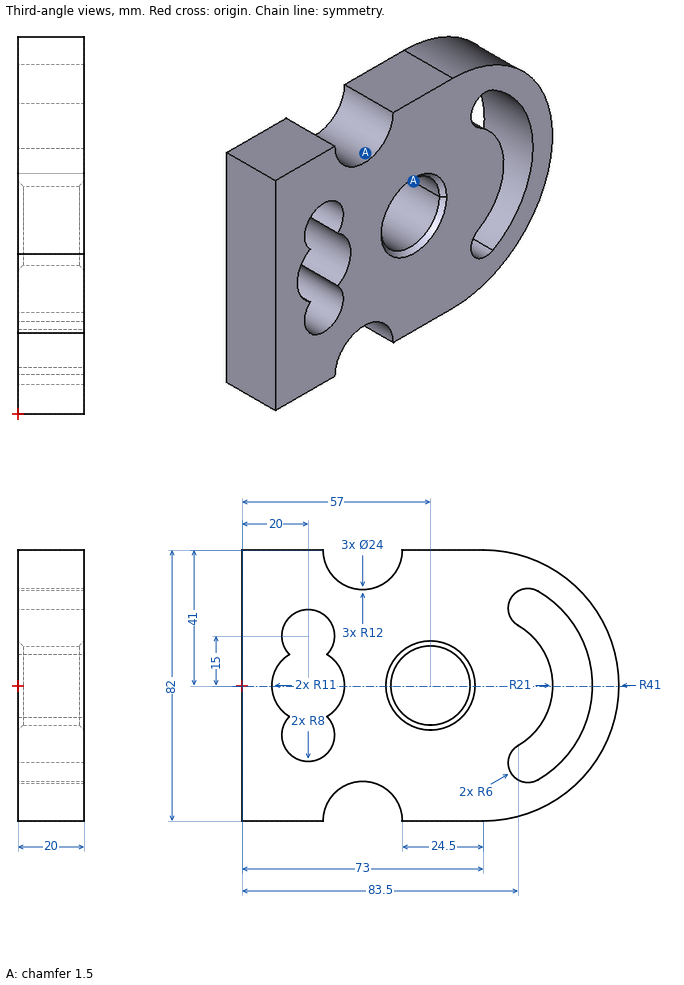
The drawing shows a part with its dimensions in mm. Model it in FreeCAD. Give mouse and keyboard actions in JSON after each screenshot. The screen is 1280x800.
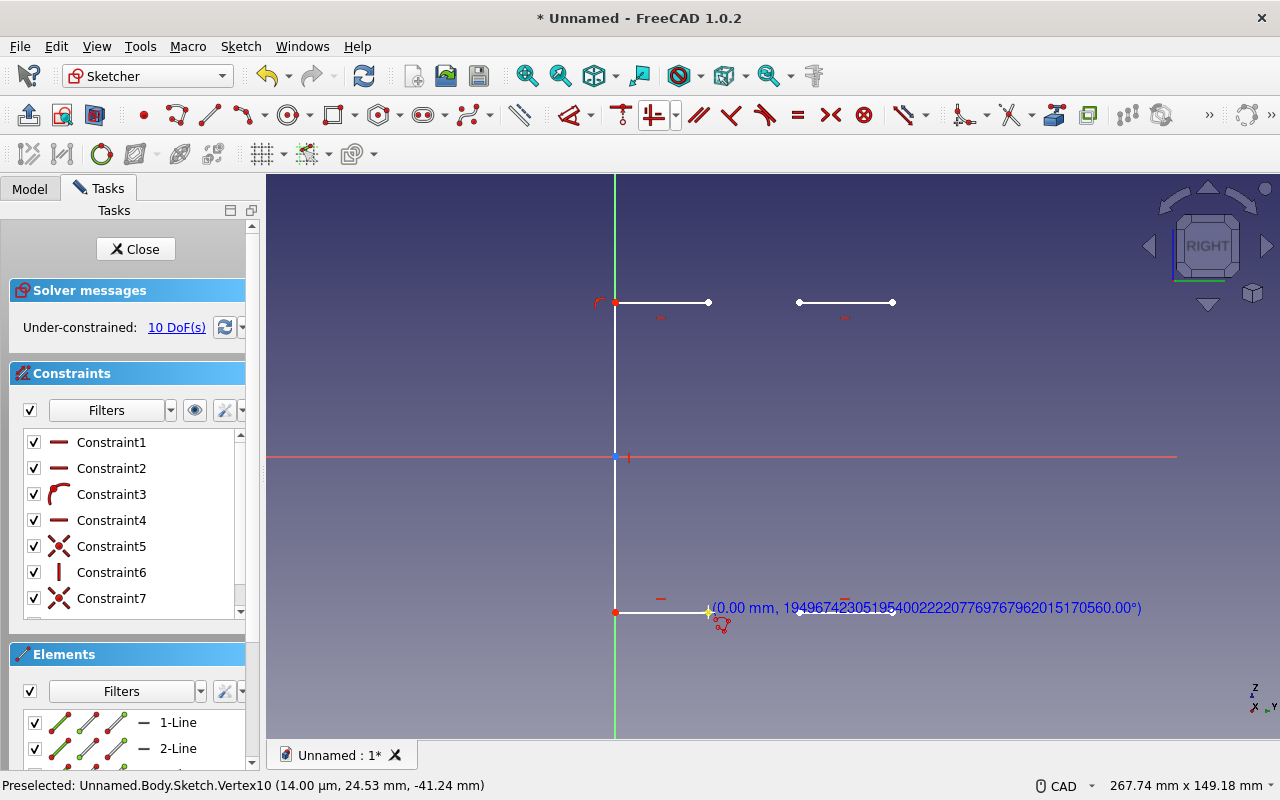
{"action": "key", "text": "g 3 a"}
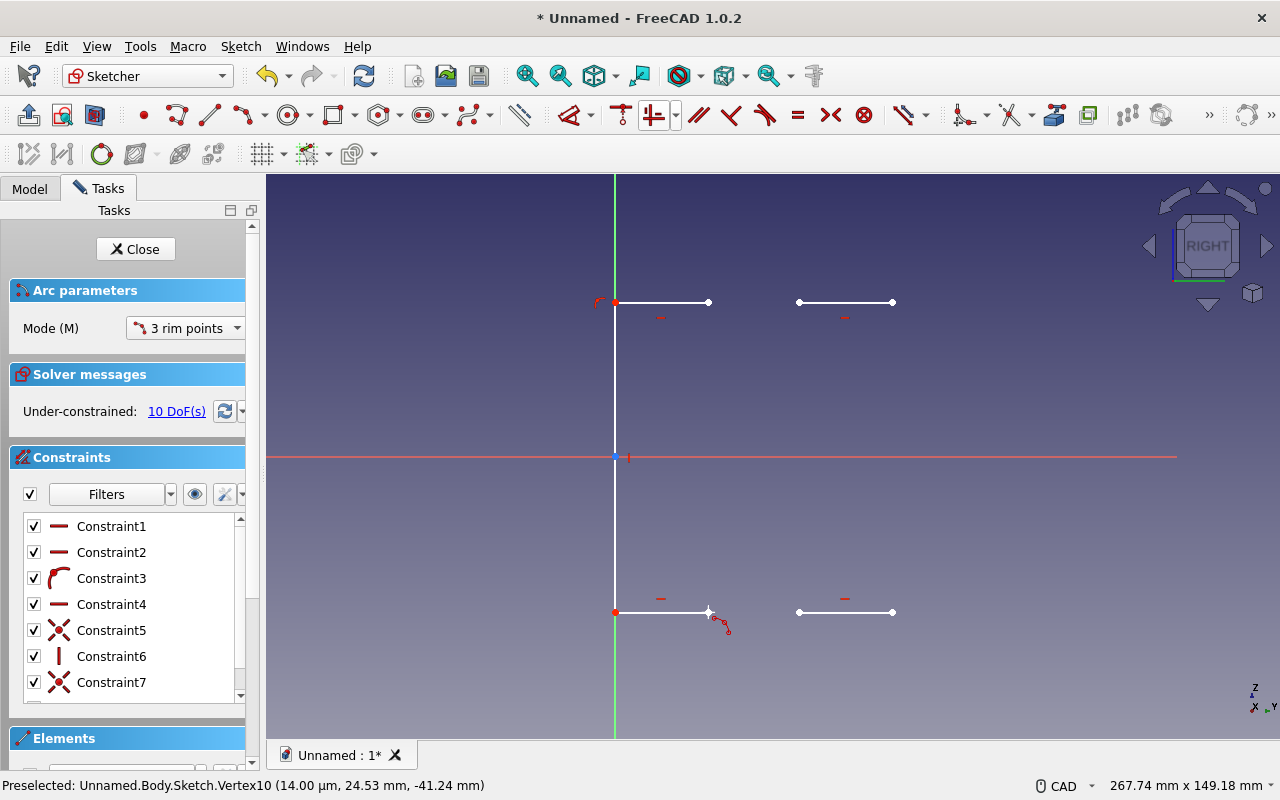
{"action": "left_click", "coordinate": [892, 613]}
{"action": "left_click", "coordinate": [892, 303]}
{"action": "left_click", "coordinate": [1039, 505]}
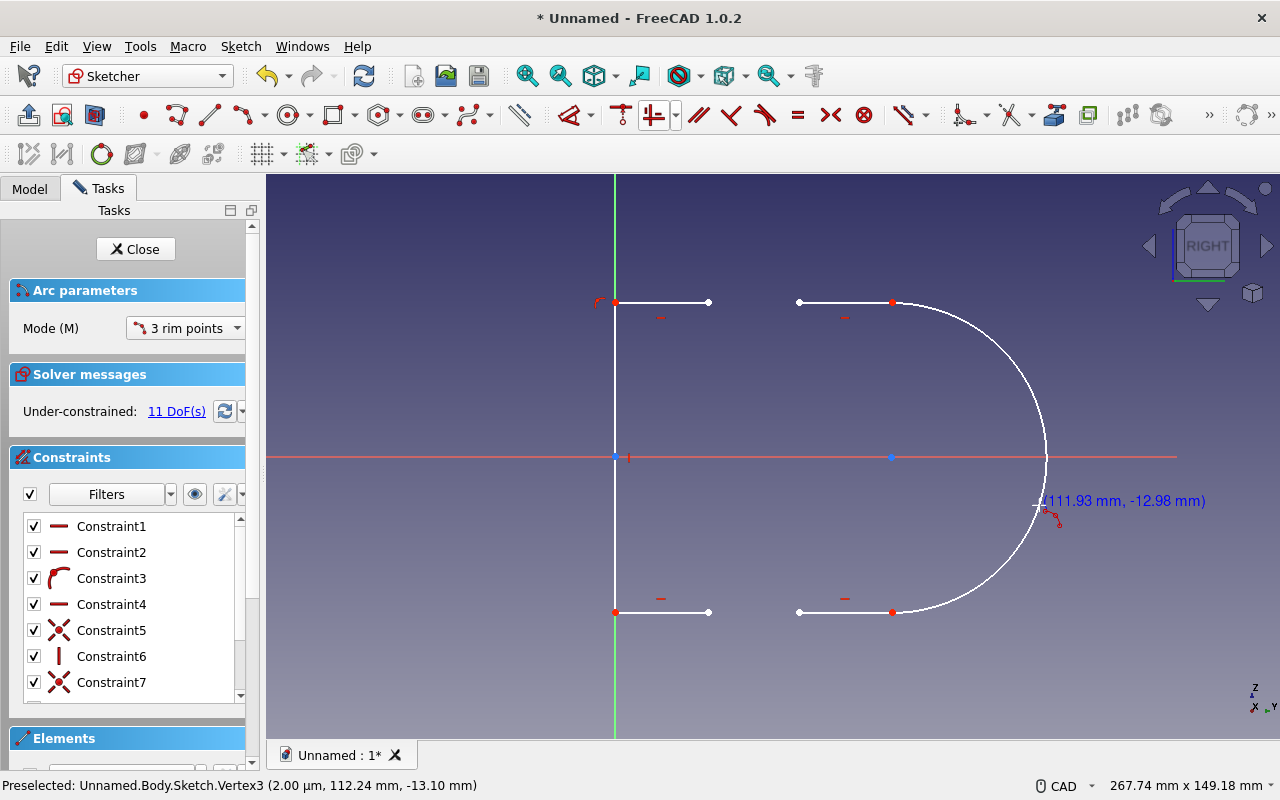
{"action": "left_click", "coordinate": [799, 303]}
{"action": "left_click", "coordinate": [708, 303]}
{"action": "left_click", "coordinate": [753, 347]}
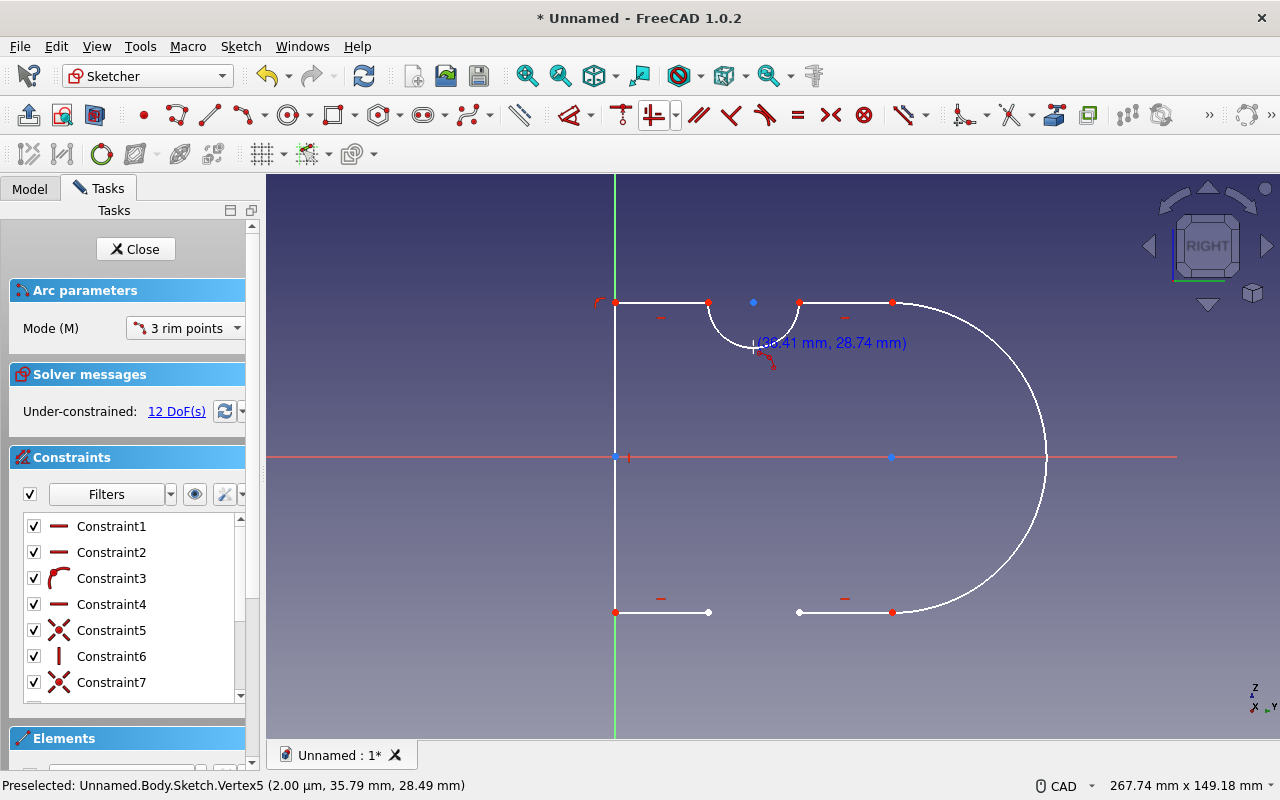
{"action": "left_click", "coordinate": [708, 613]}
{"action": "left_click", "coordinate": [799, 613]}
{"action": "left_click", "coordinate": [753, 567]}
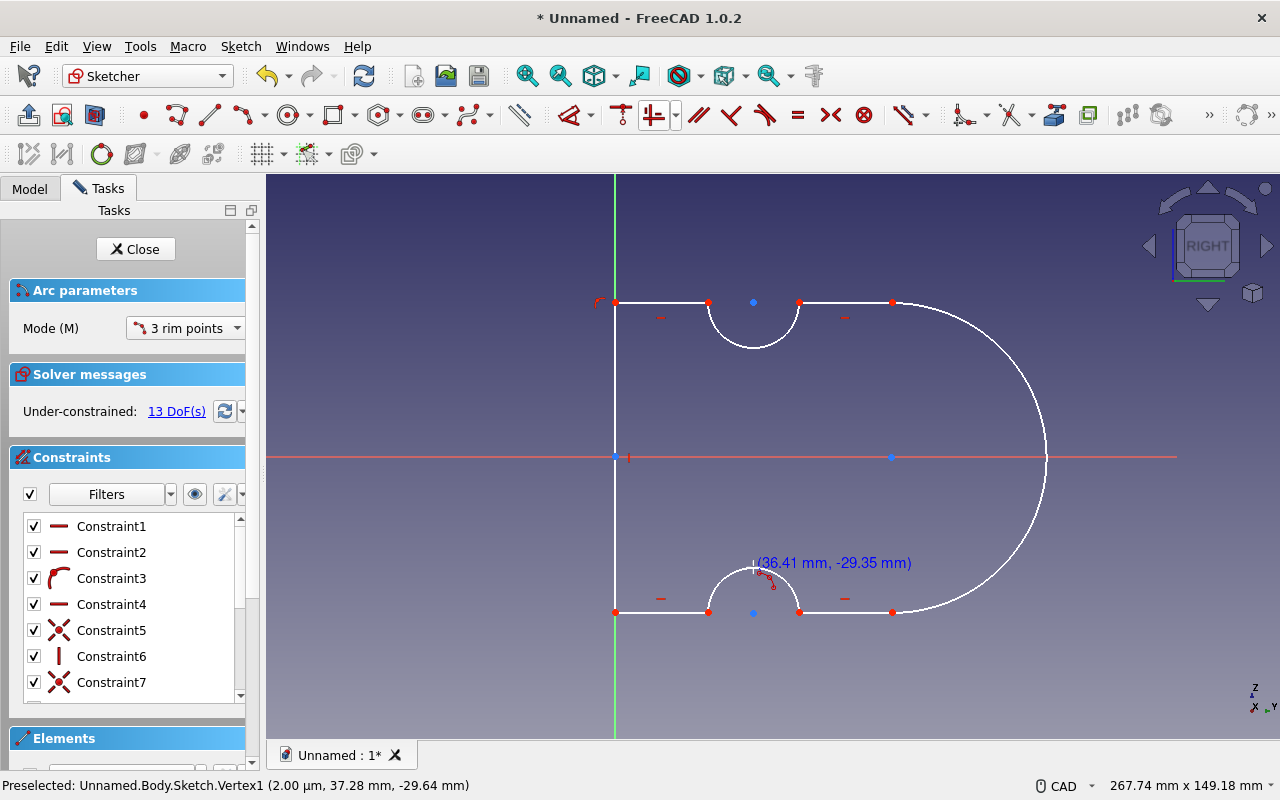
{"action": "left_click", "coordinate": [669, 492]}
{"action": "left_click", "coordinate": [669, 421]}
{"action": "left_click", "coordinate": [653, 440]}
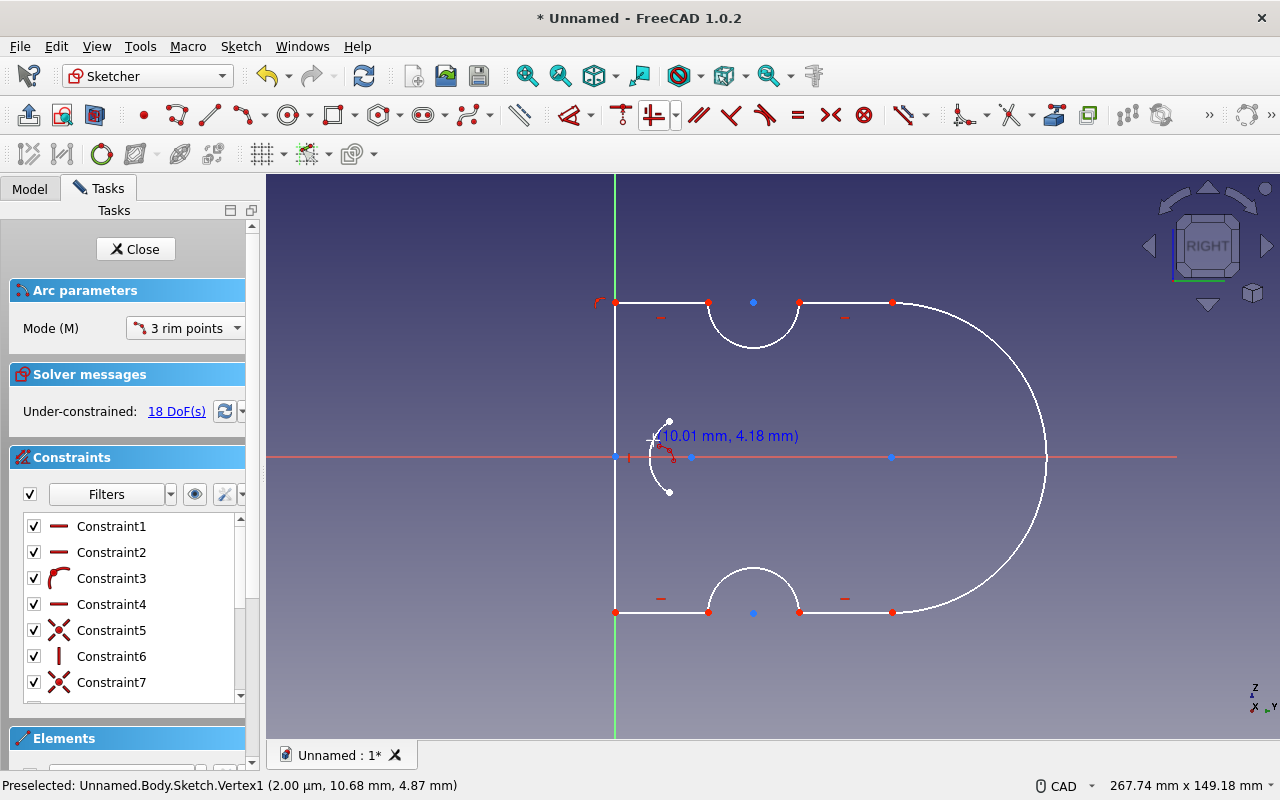
{"action": "left_click", "coordinate": [669, 422]}
{"action": "left_click", "coordinate": [712, 421]}
{"action": "left_click", "coordinate": [691, 370]}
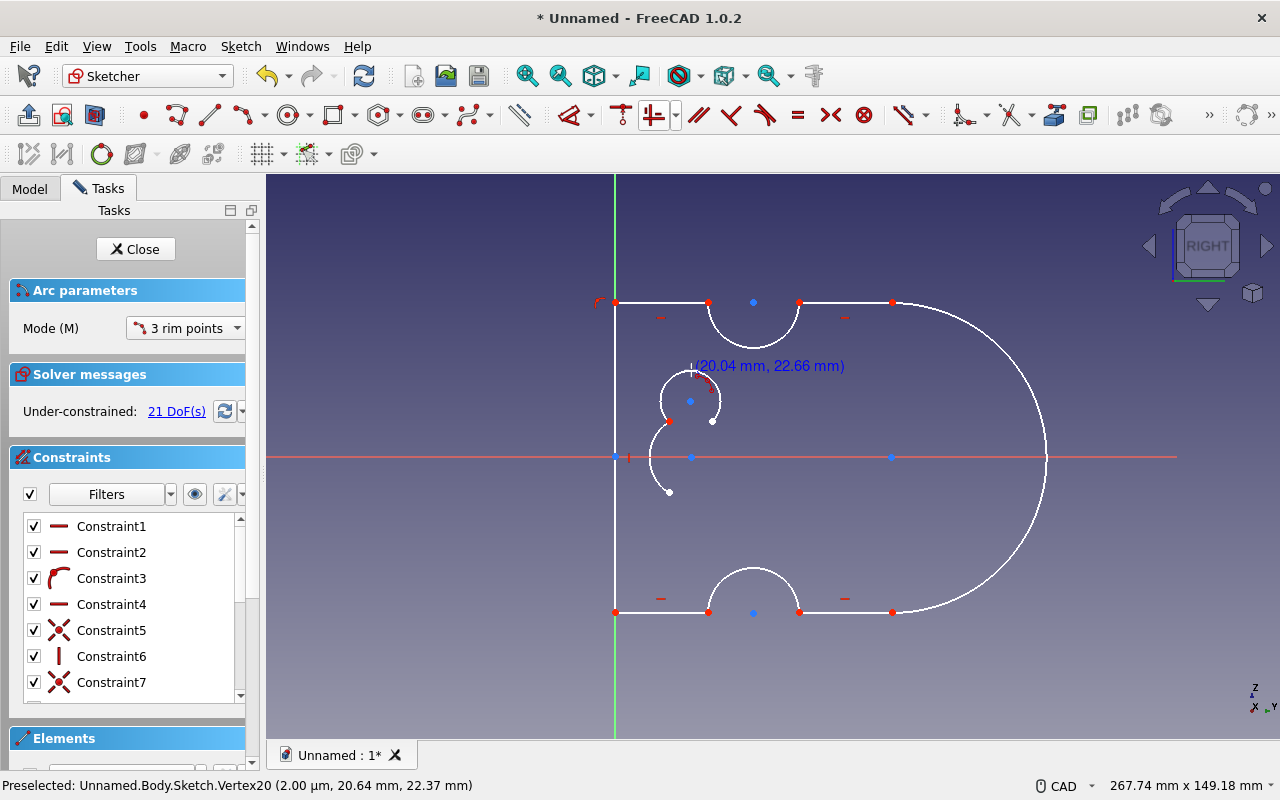
{"action": "left_click", "coordinate": [712, 422]}
{"action": "left_click", "coordinate": [712, 492]}
{"action": "left_click", "coordinate": [729, 473]}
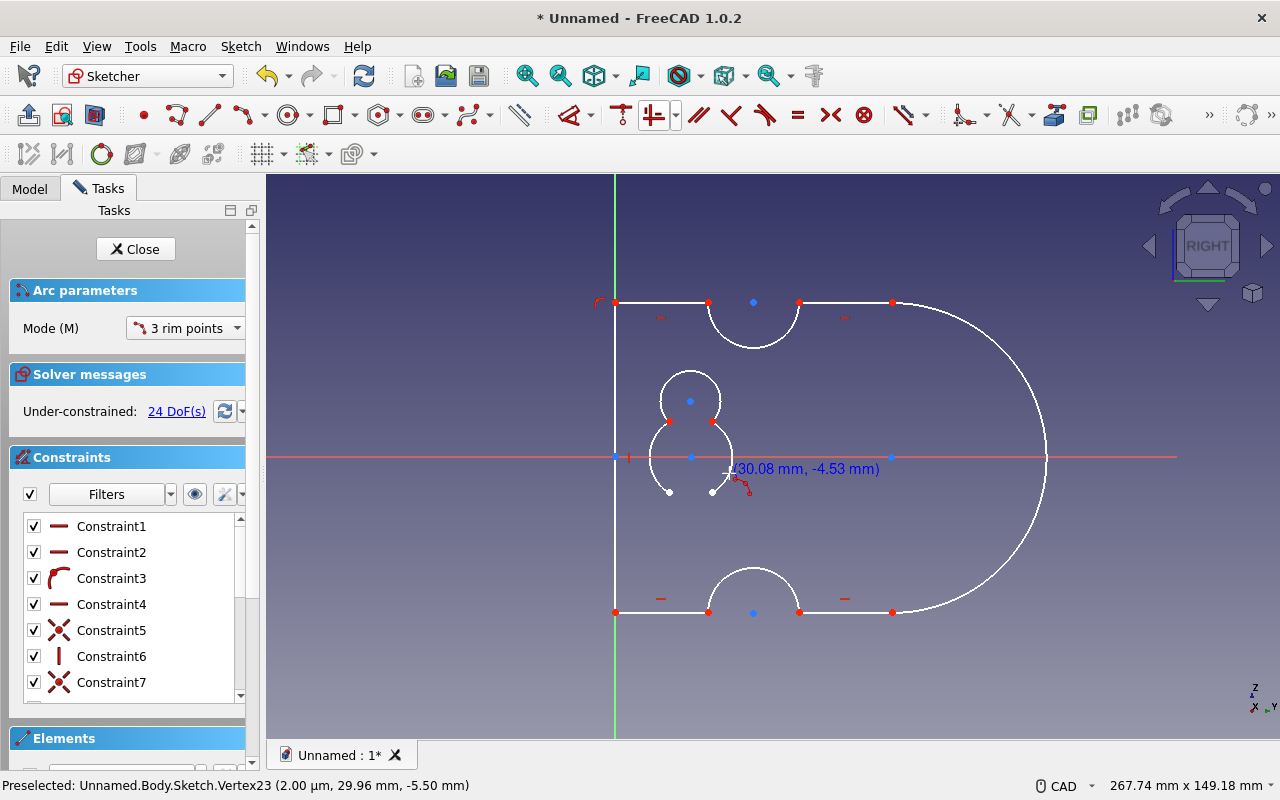
{"action": "left_click", "coordinate": [712, 493]}
{"action": "left_click", "coordinate": [669, 493]}
{"action": "left_click", "coordinate": [691, 544]}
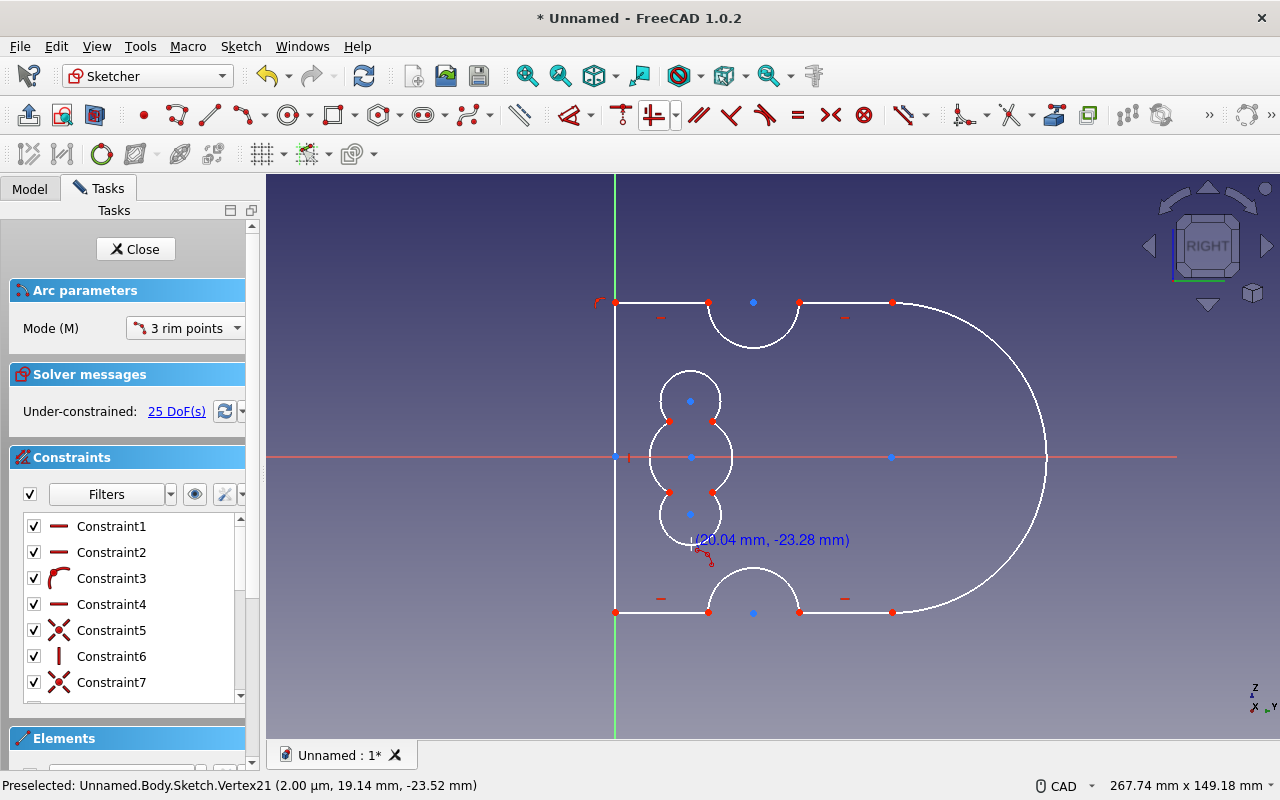
{"action": "left_click", "coordinate": [931, 526]}
{"action": "left_click", "coordinate": [931, 388]}
{"action": "left_click", "coordinate": [969, 473]}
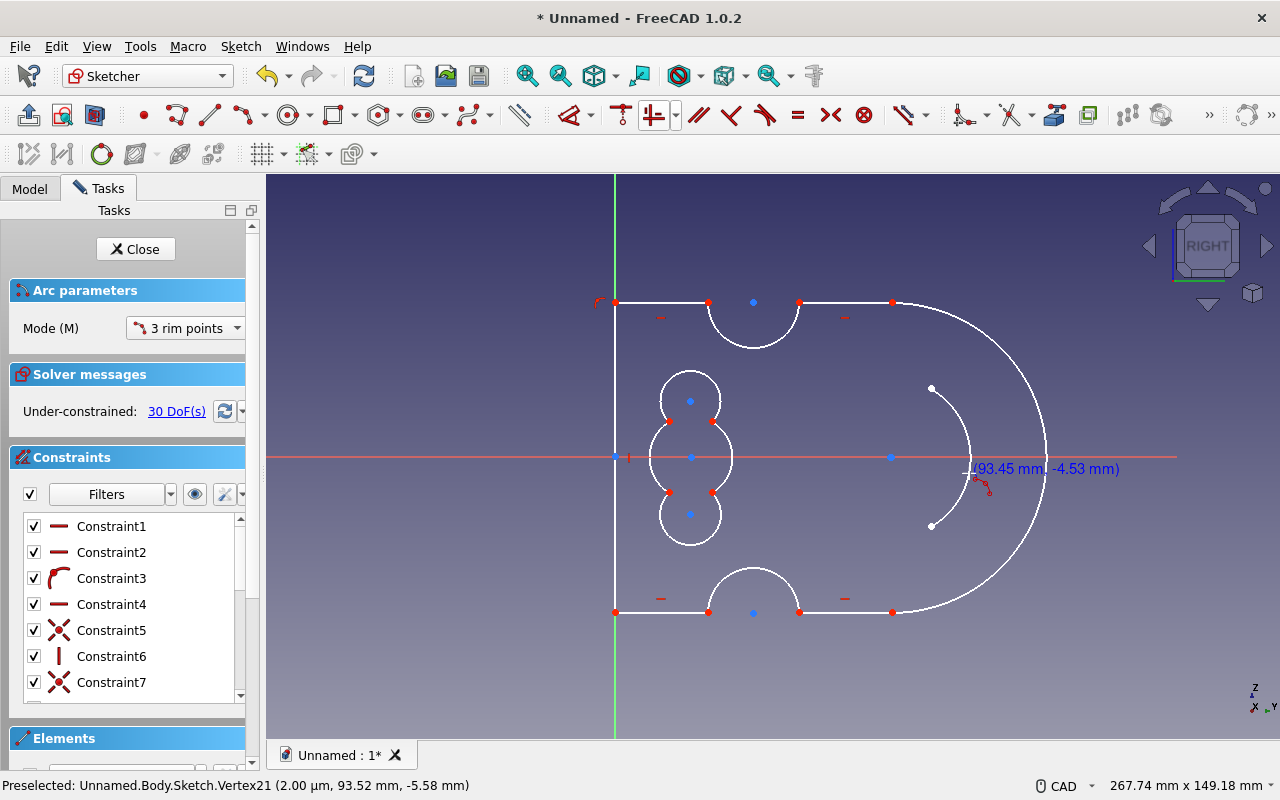
{"action": "left_click", "coordinate": [931, 389]}
{"action": "left_click", "coordinate": [954, 349]}
{"action": "left_click", "coordinate": [923, 357]}